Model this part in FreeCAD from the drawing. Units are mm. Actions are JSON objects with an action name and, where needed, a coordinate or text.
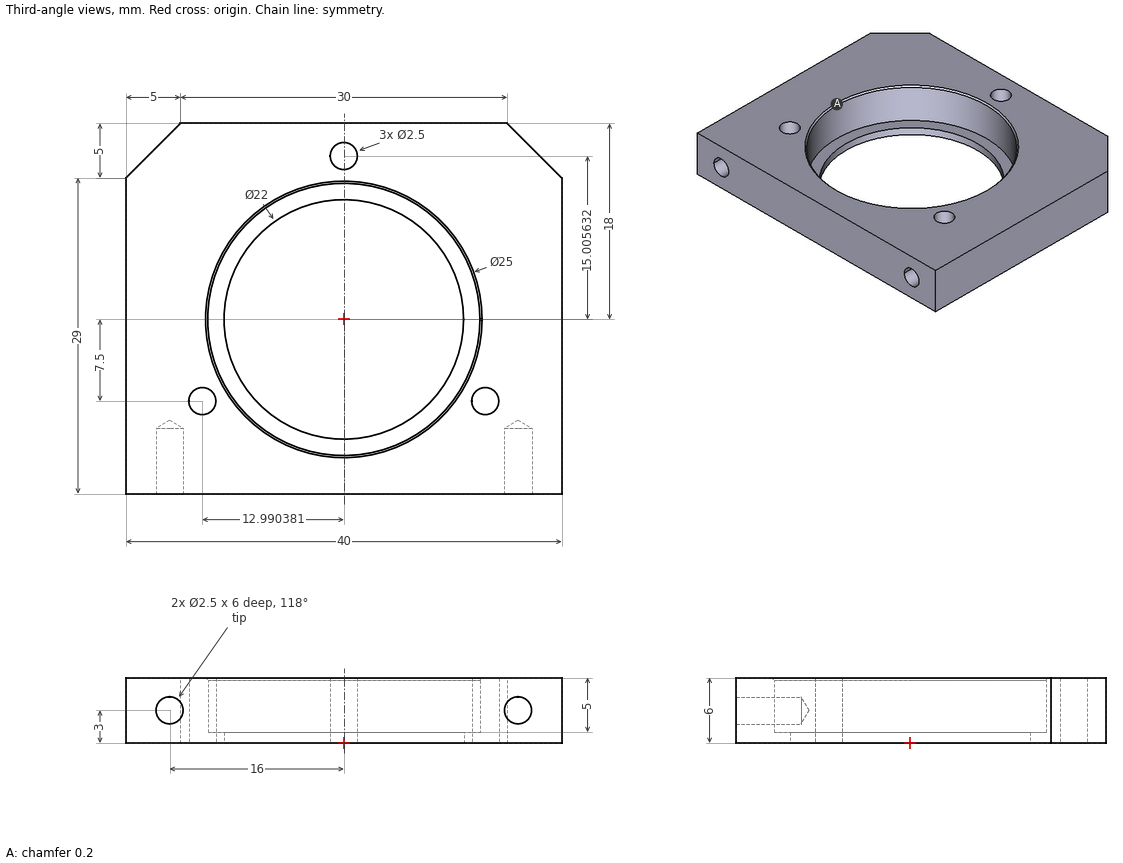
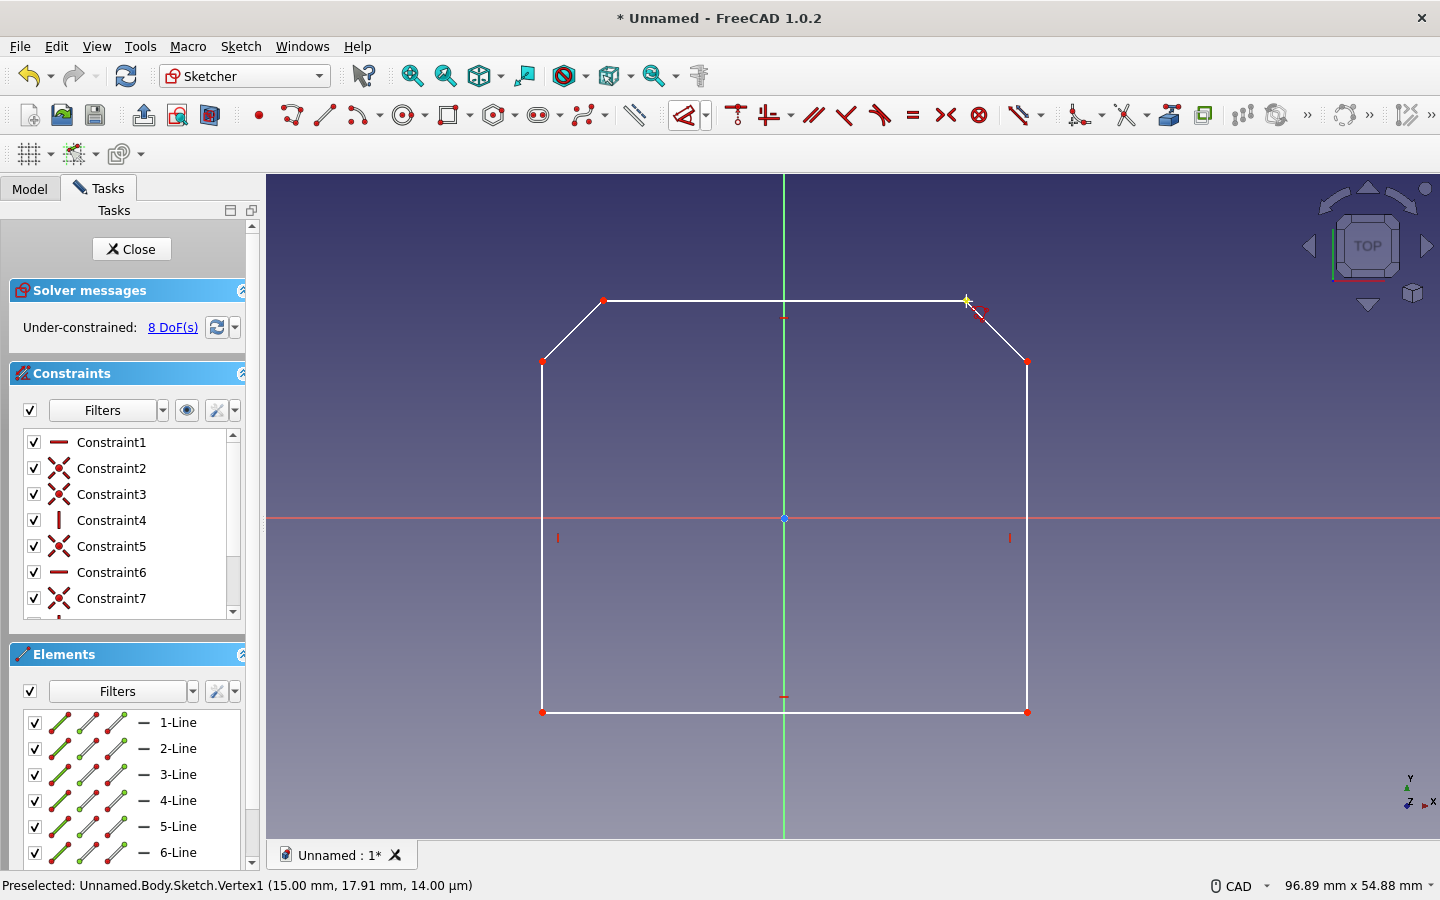
{"action": "left_click", "coordinate": [402, 116]}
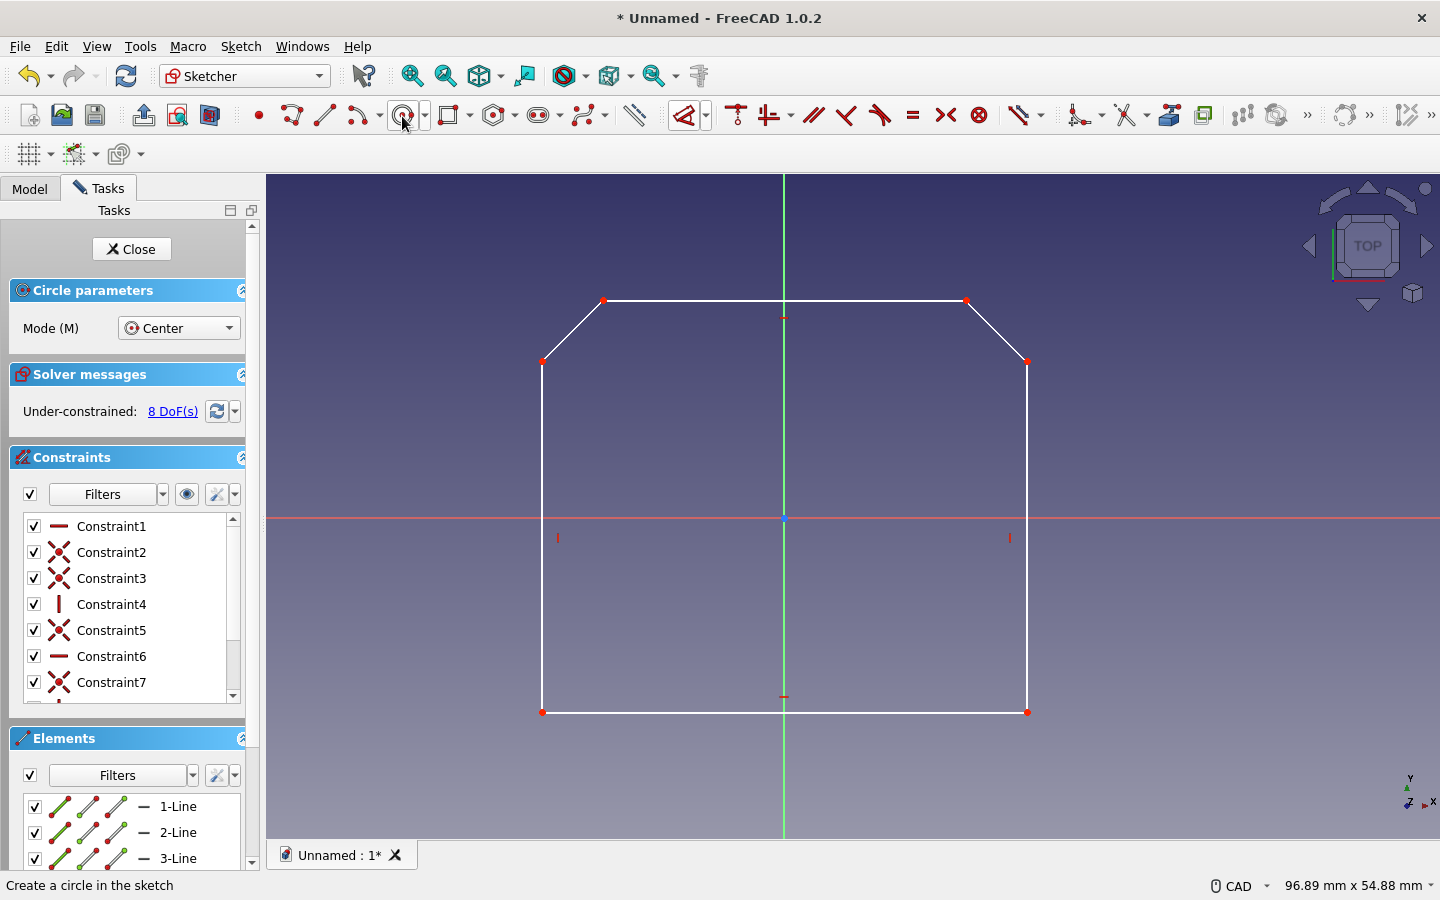
{"action": "left_click", "coordinate": [784, 518]}
{"action": "left_click", "coordinate": [879, 424]}
{"action": "key", "text": "Escape"}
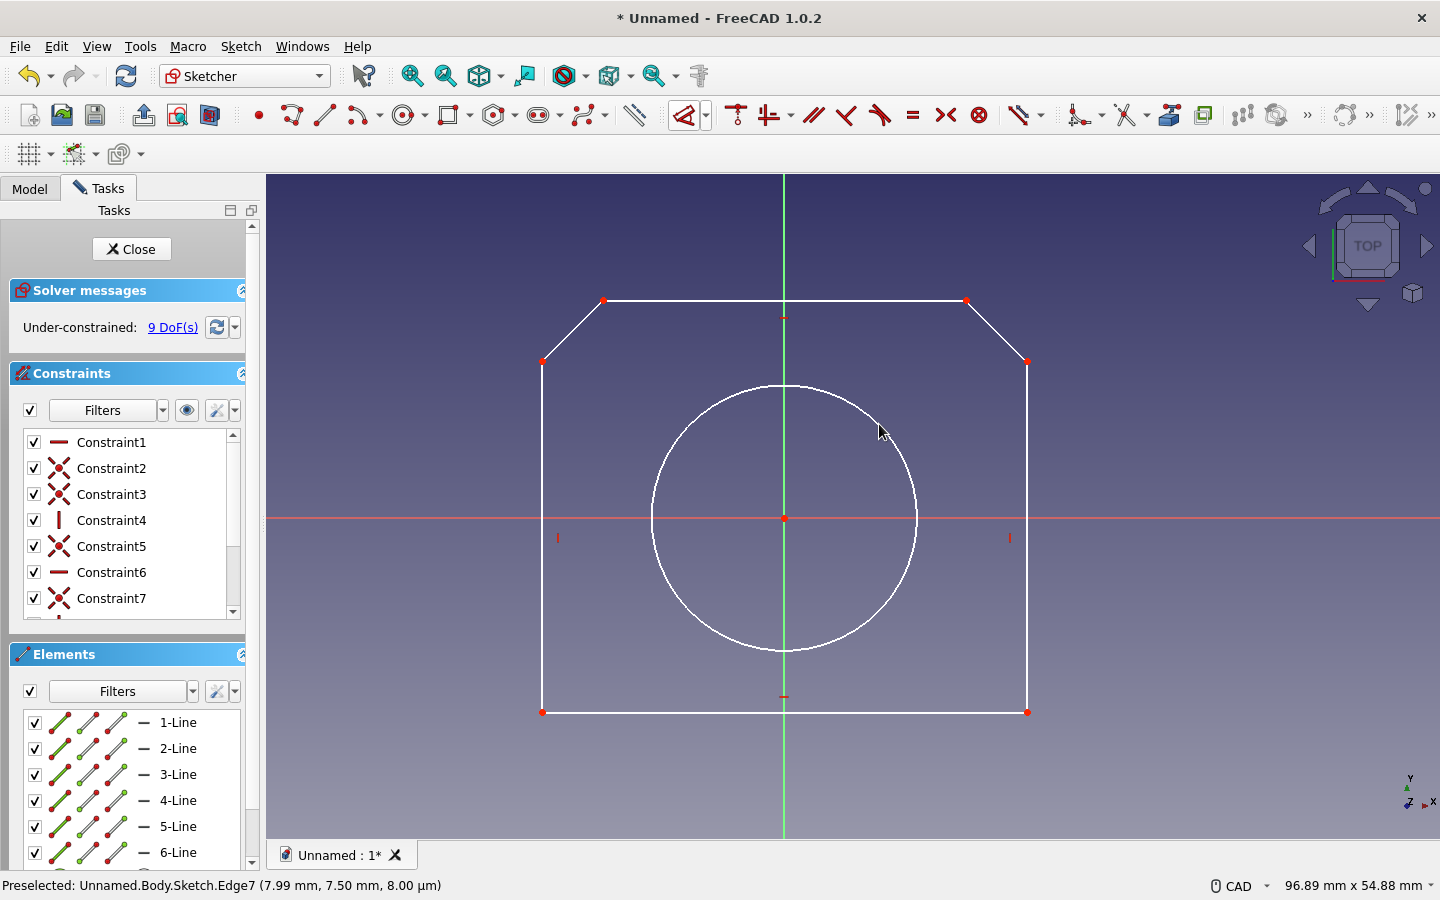
{"action": "left_click", "coordinate": [542, 362]}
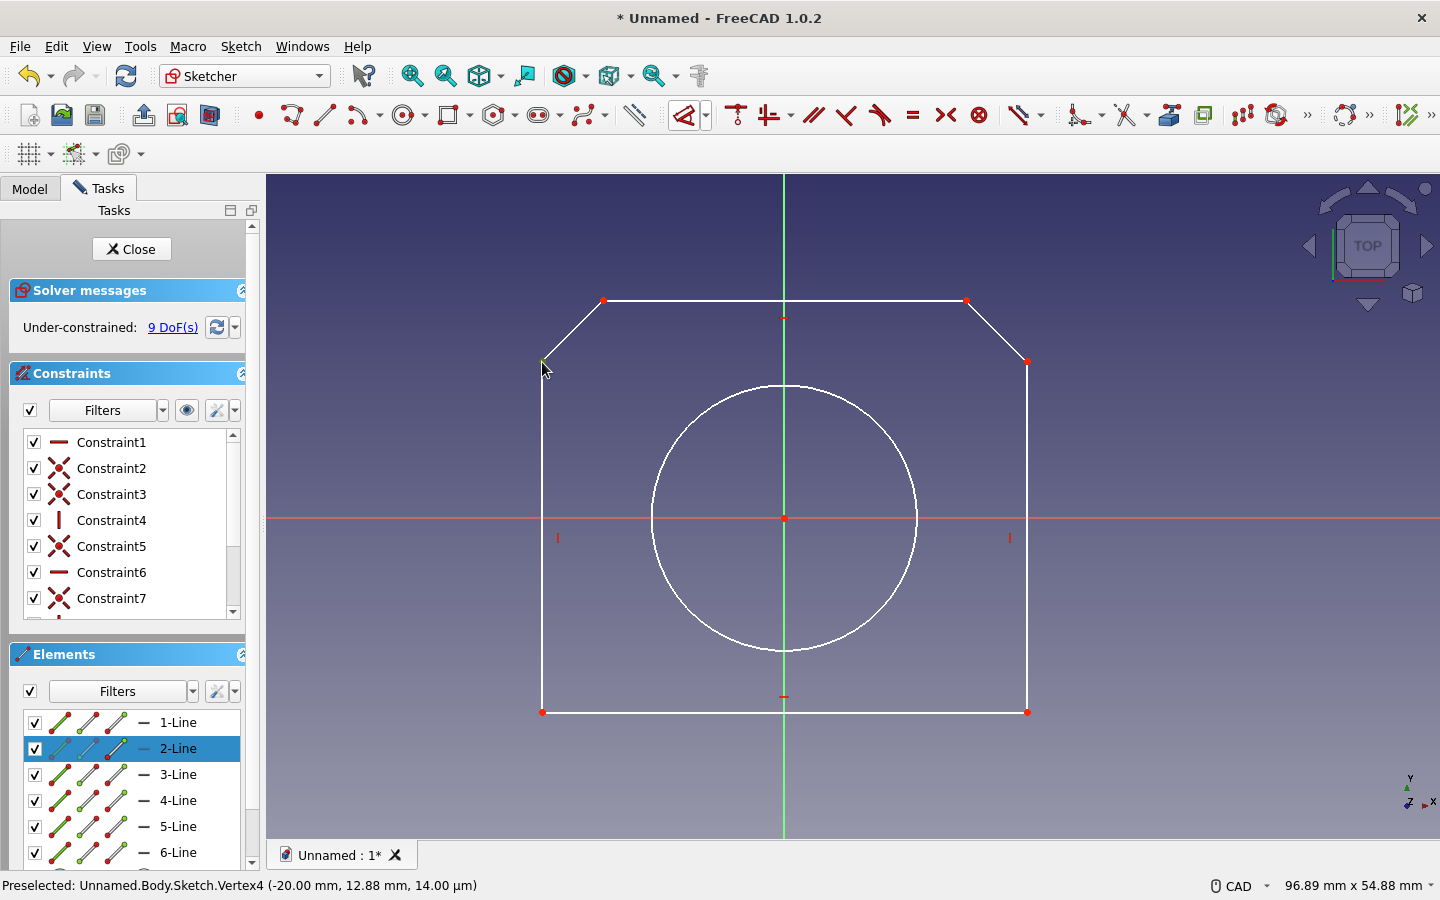
{"action": "left_click", "coordinate": [1027, 362]}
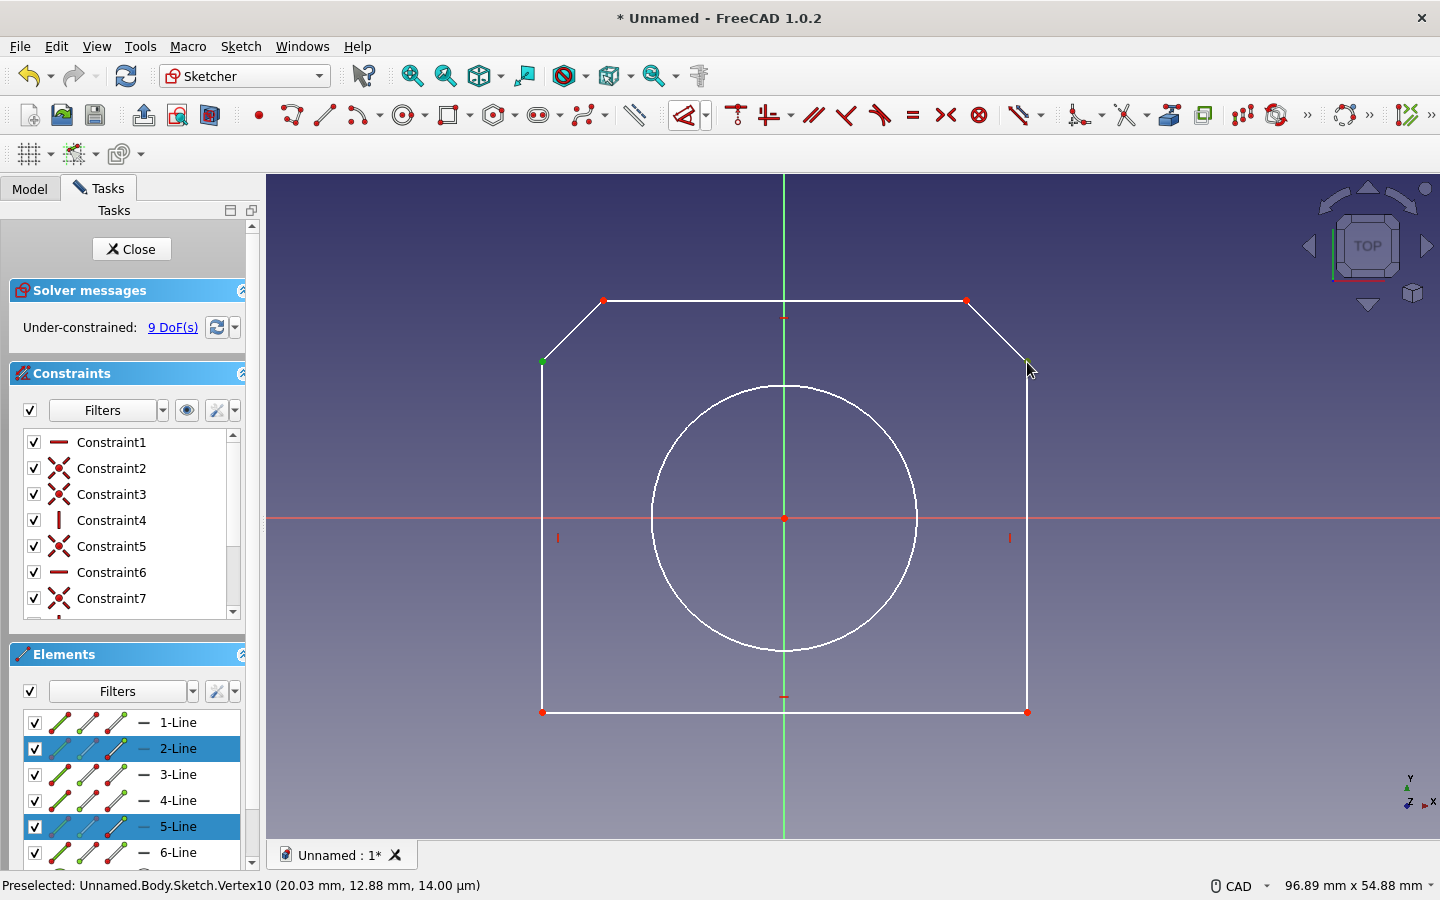
{"action": "left_click", "coordinate": [784, 768]}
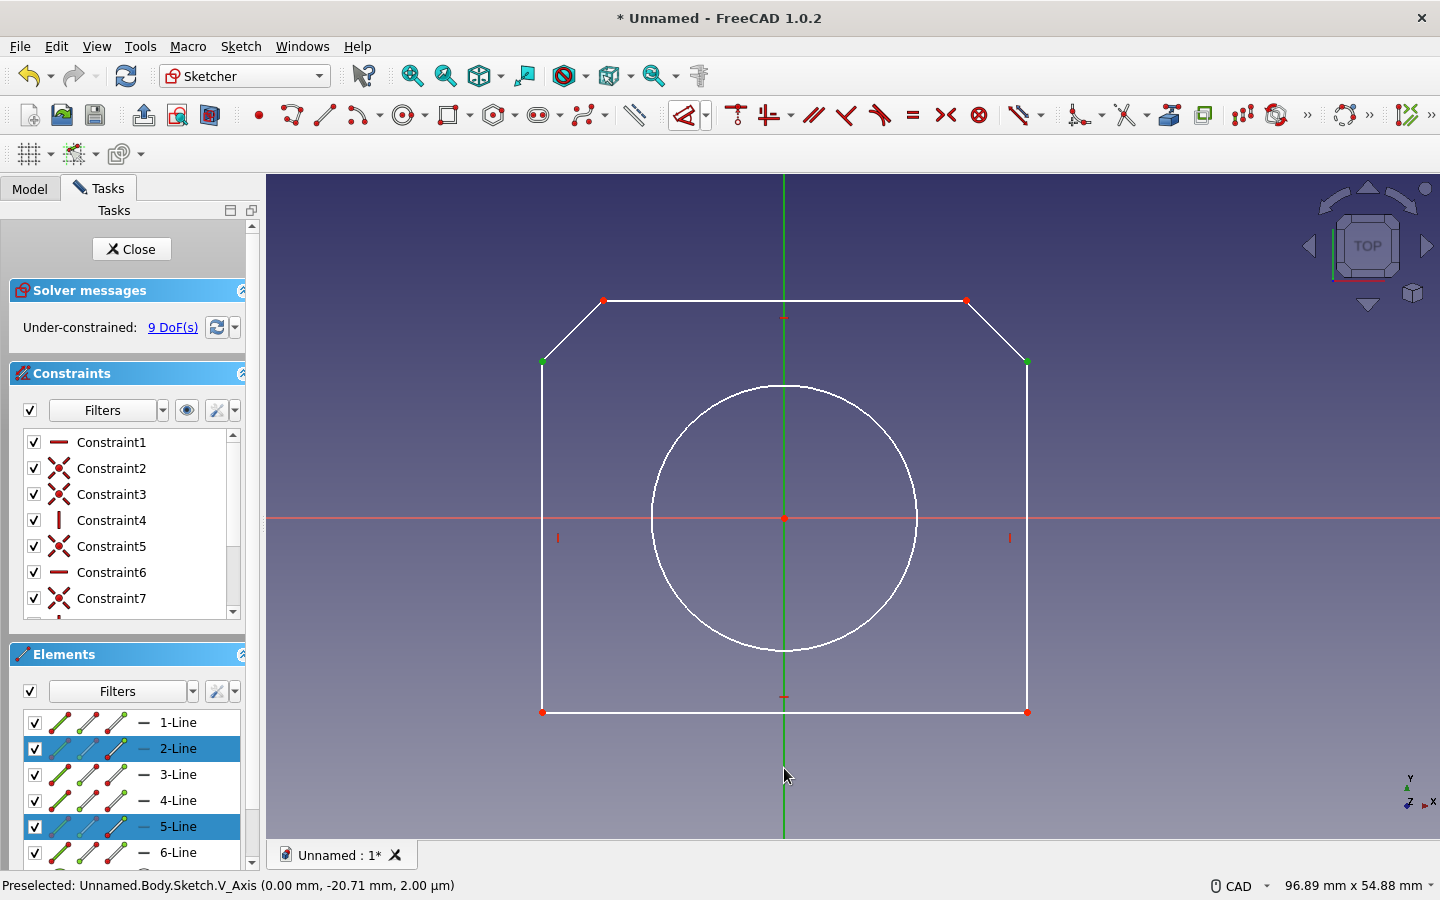
{"action": "left_click", "coordinate": [946, 116]}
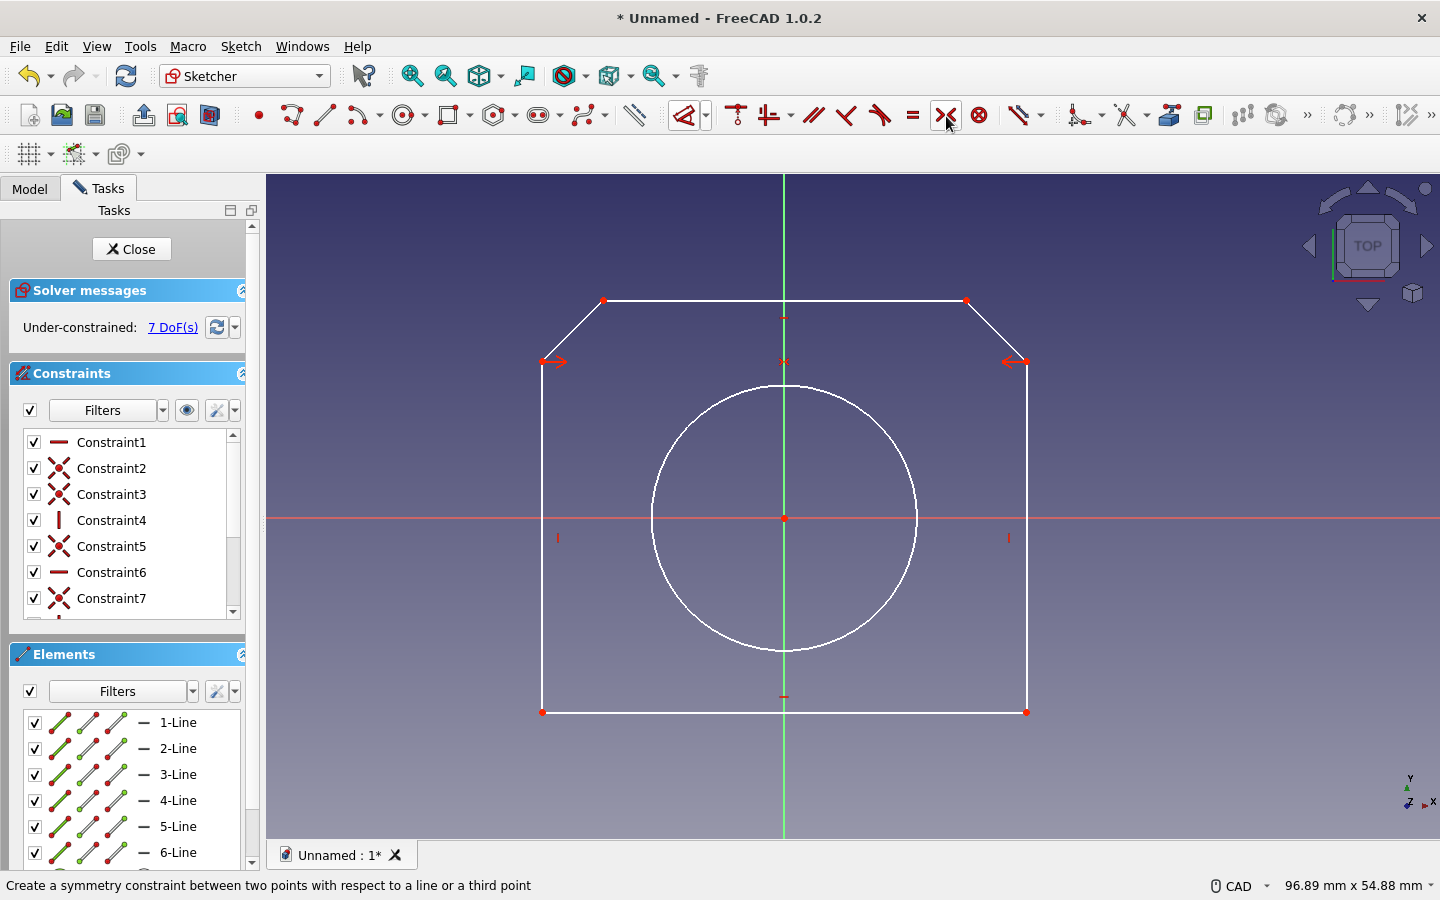
{"action": "left_click", "coordinate": [684, 116]}